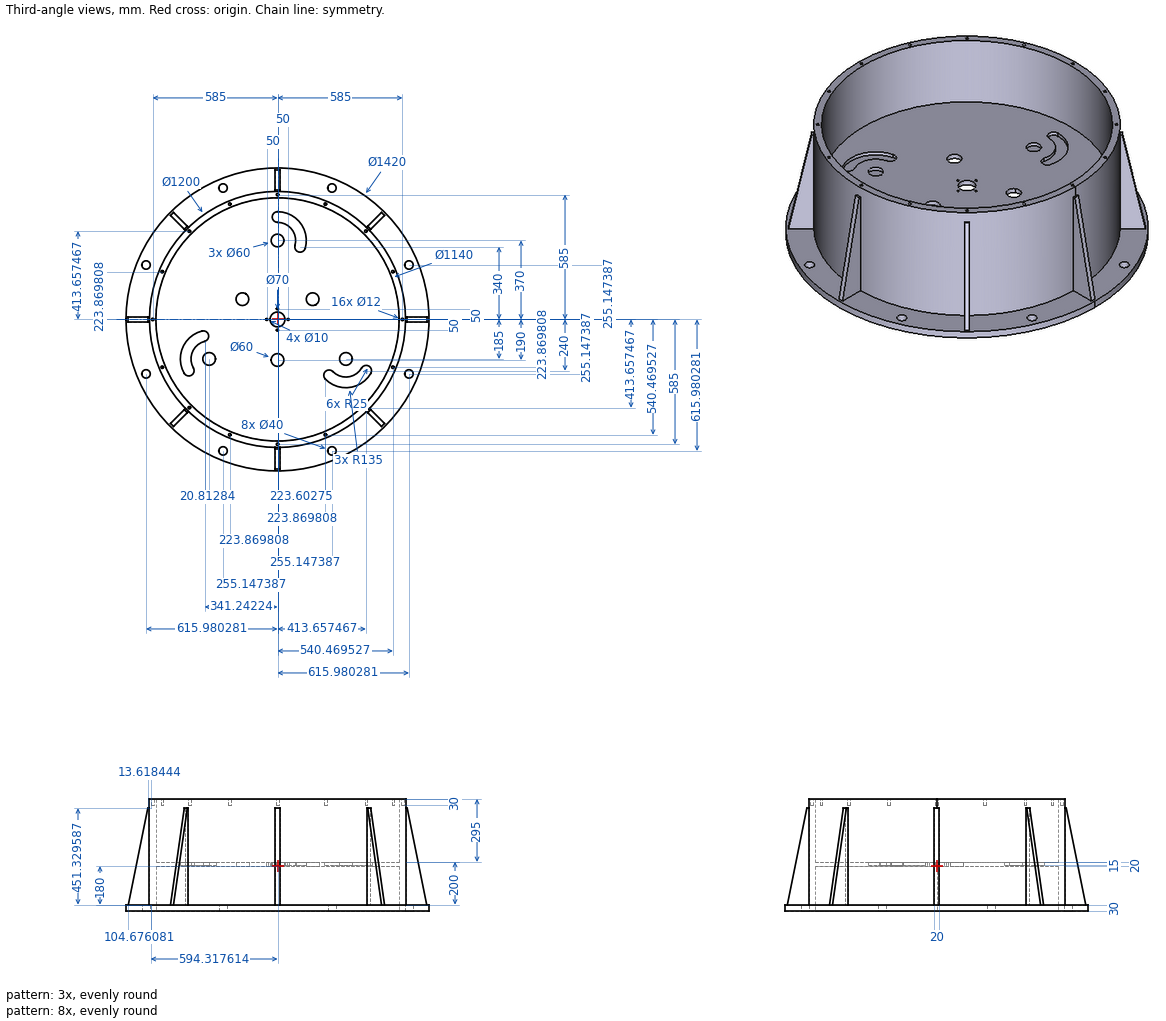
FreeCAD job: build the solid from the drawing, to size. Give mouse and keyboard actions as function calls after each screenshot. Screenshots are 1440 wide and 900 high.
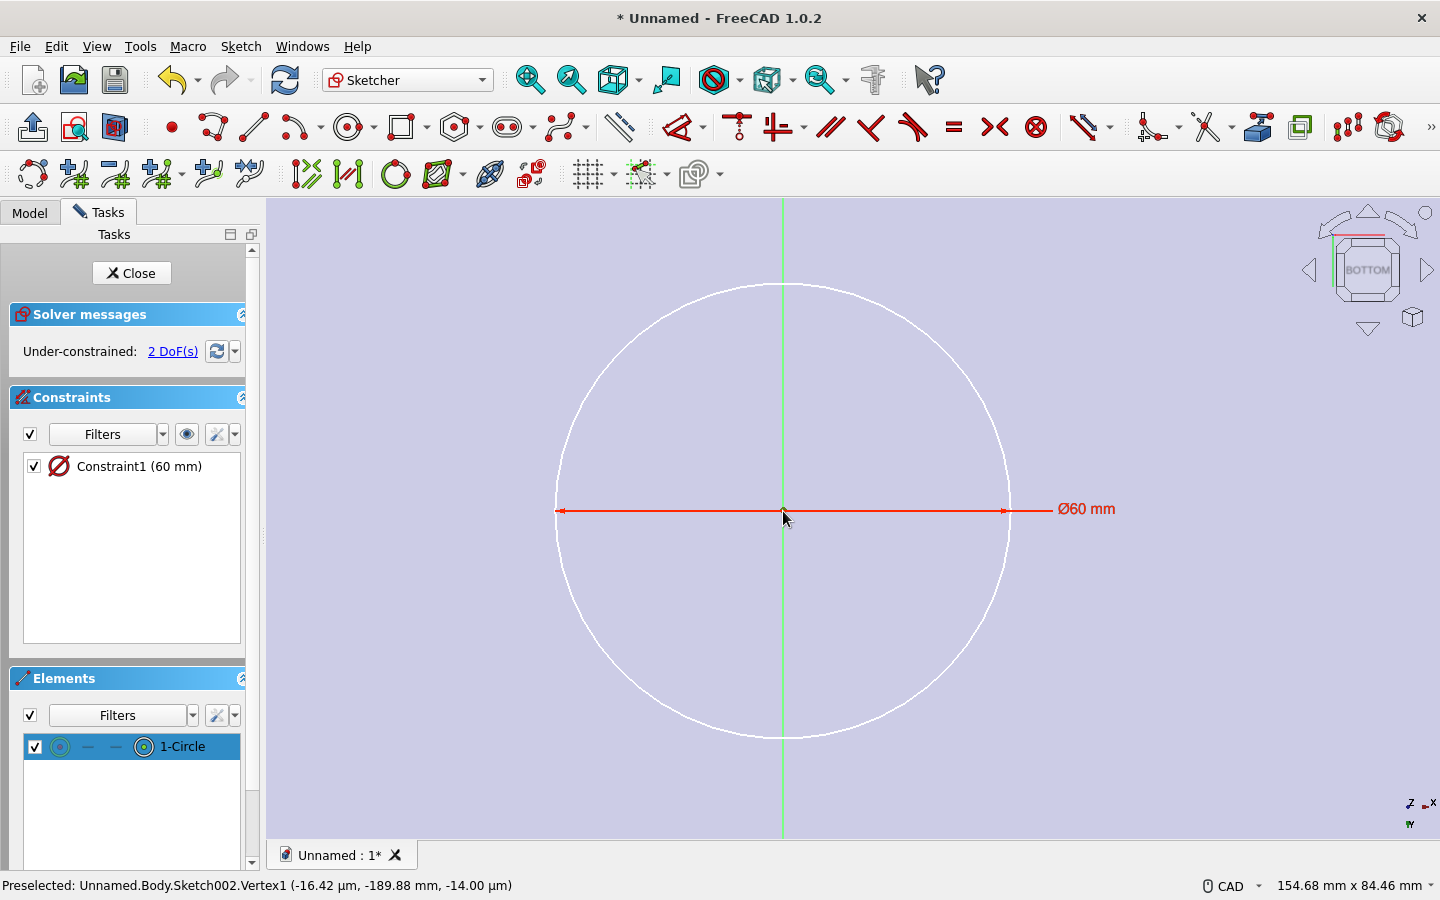
click(783, 769)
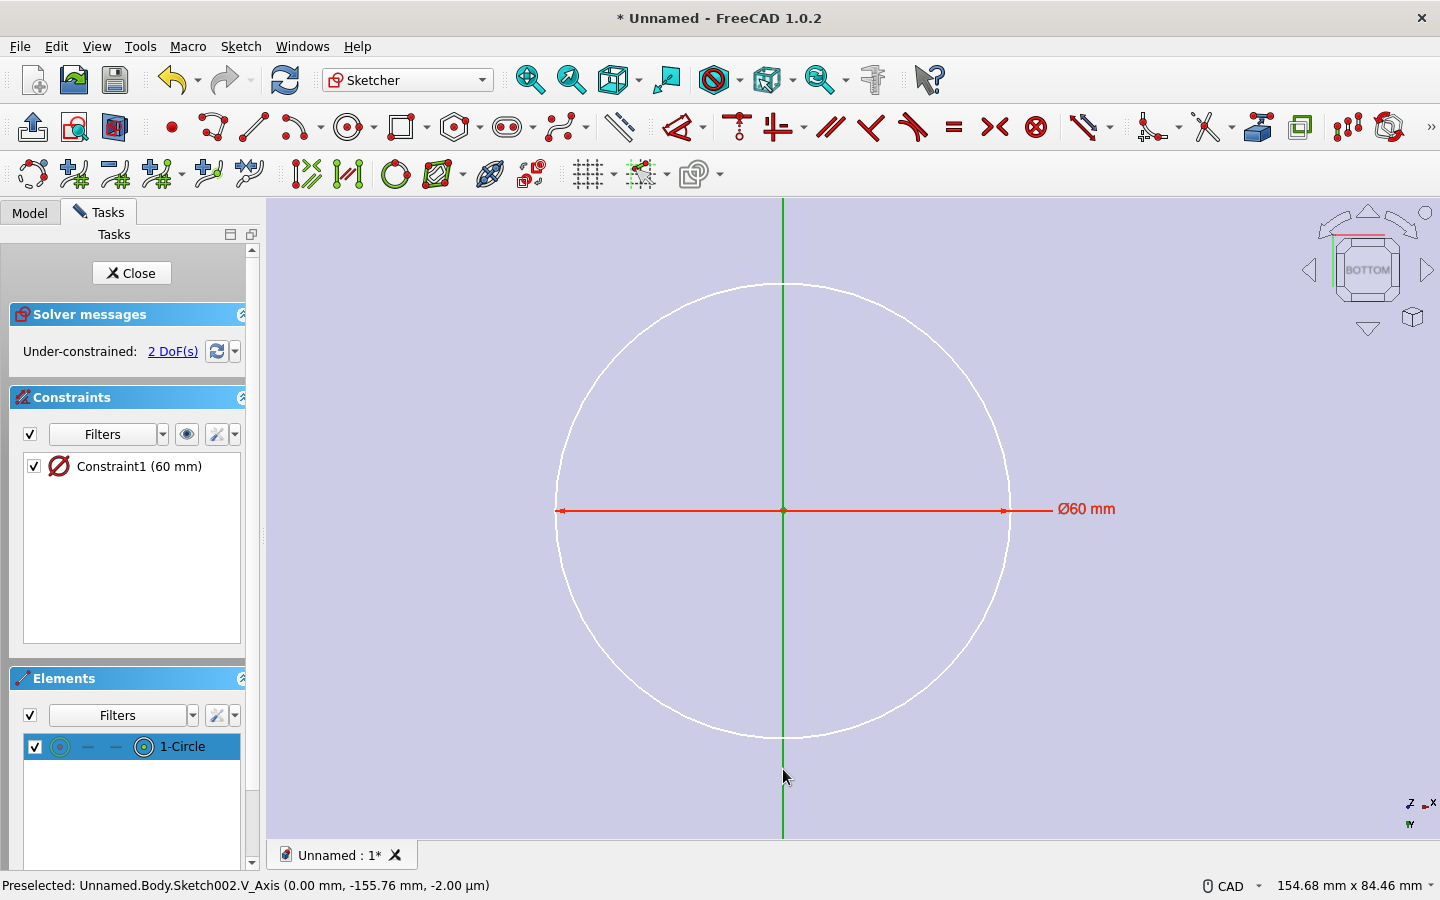
key(c)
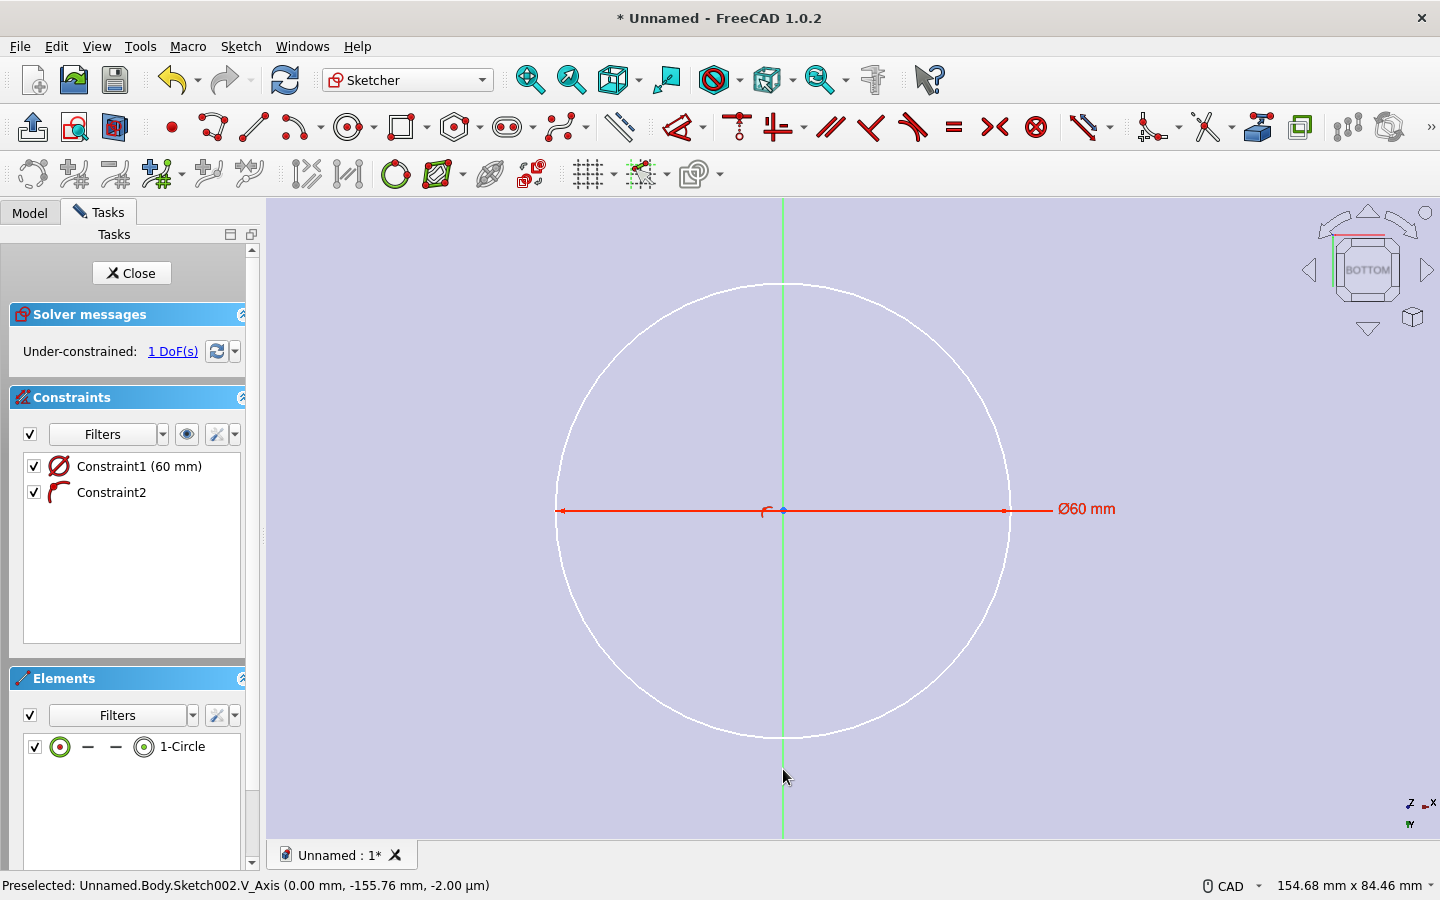
click(783, 511)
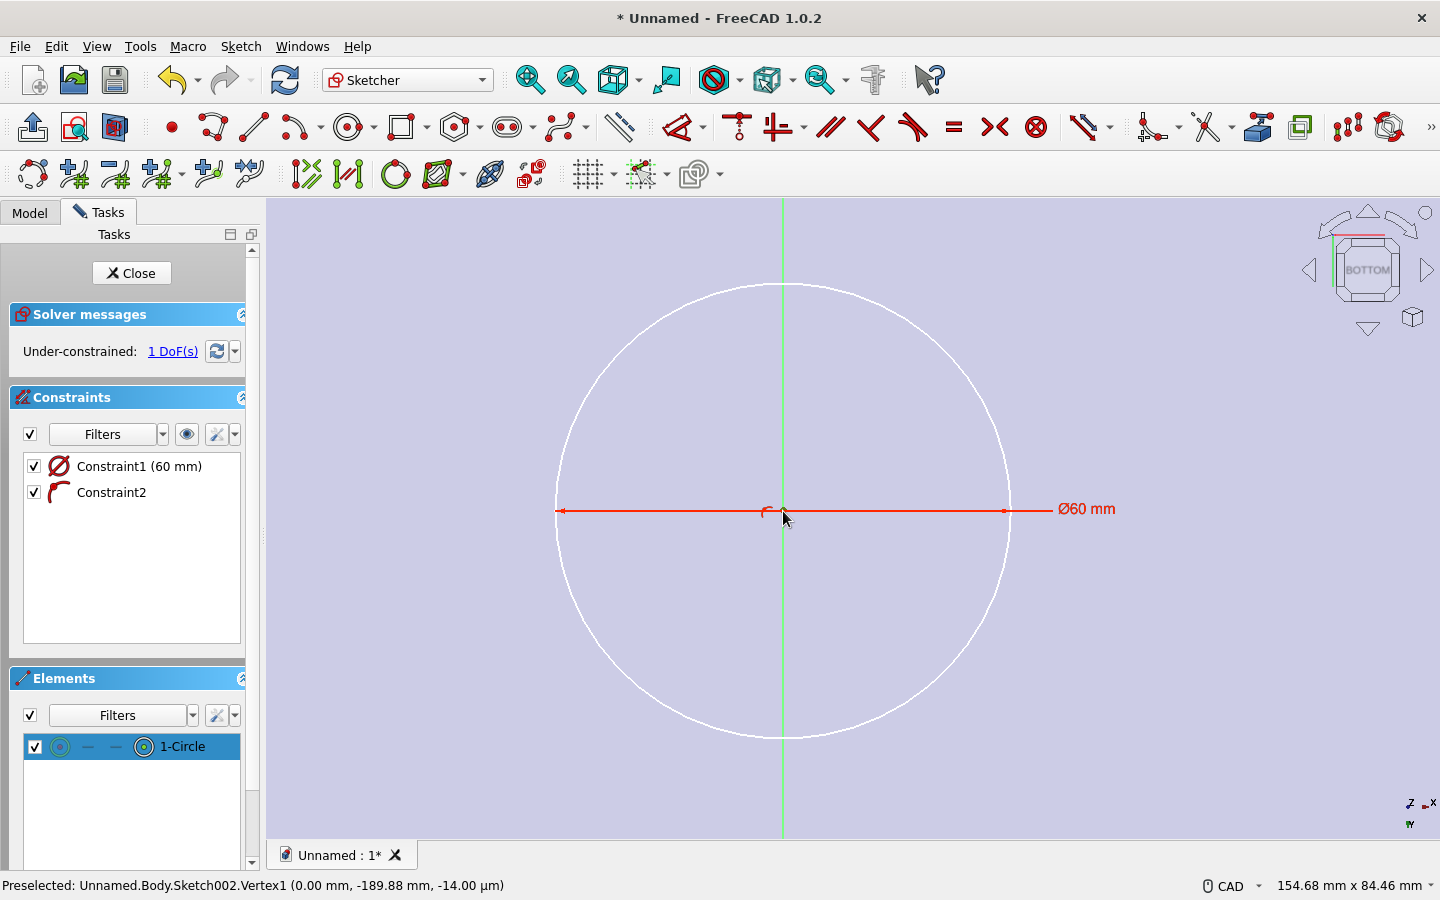
click(702, 128)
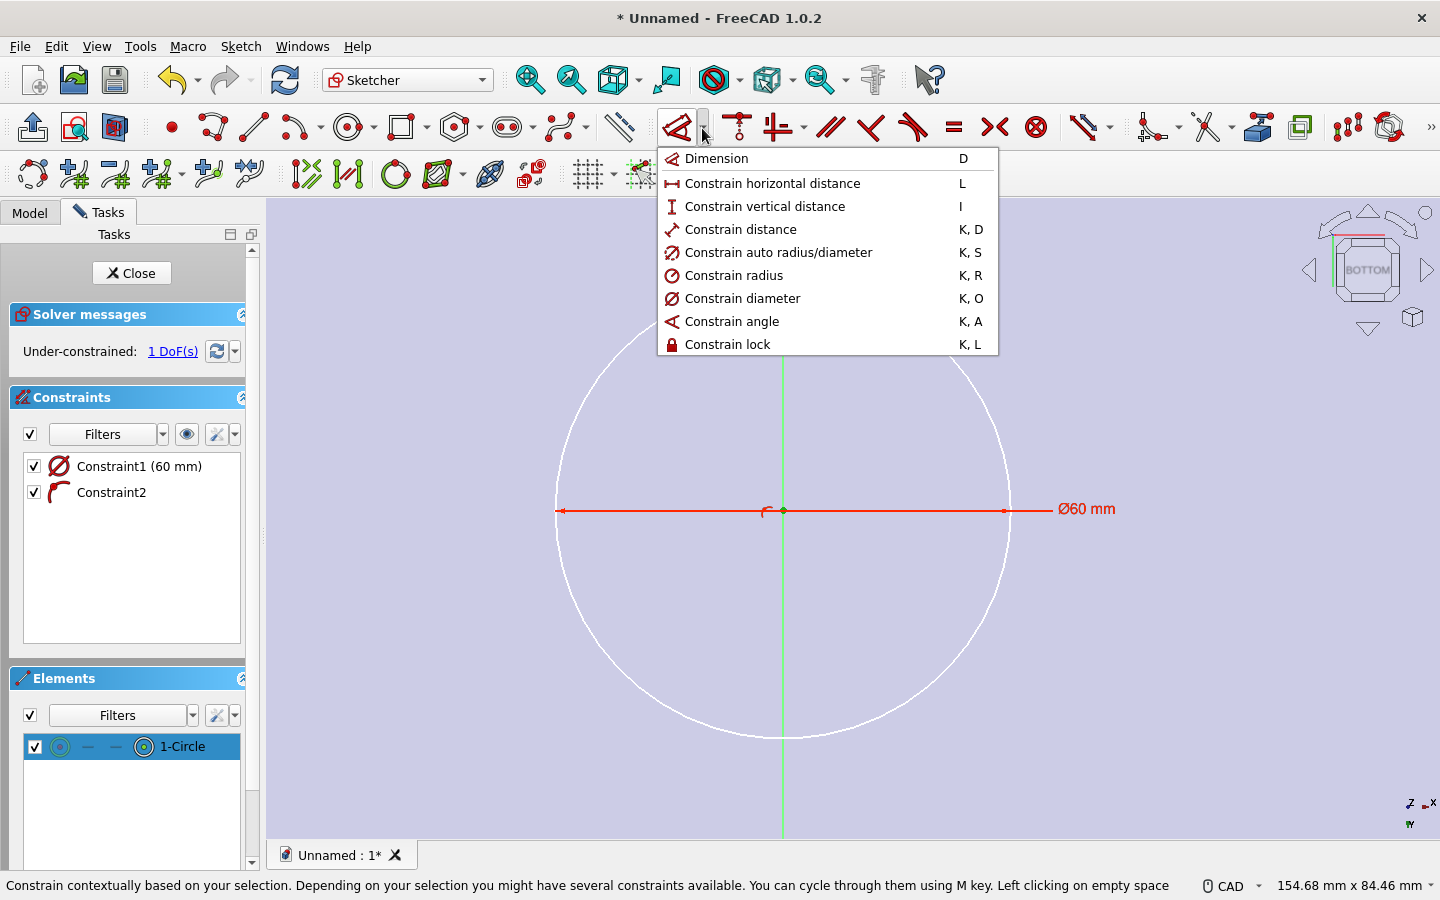
click(828, 206)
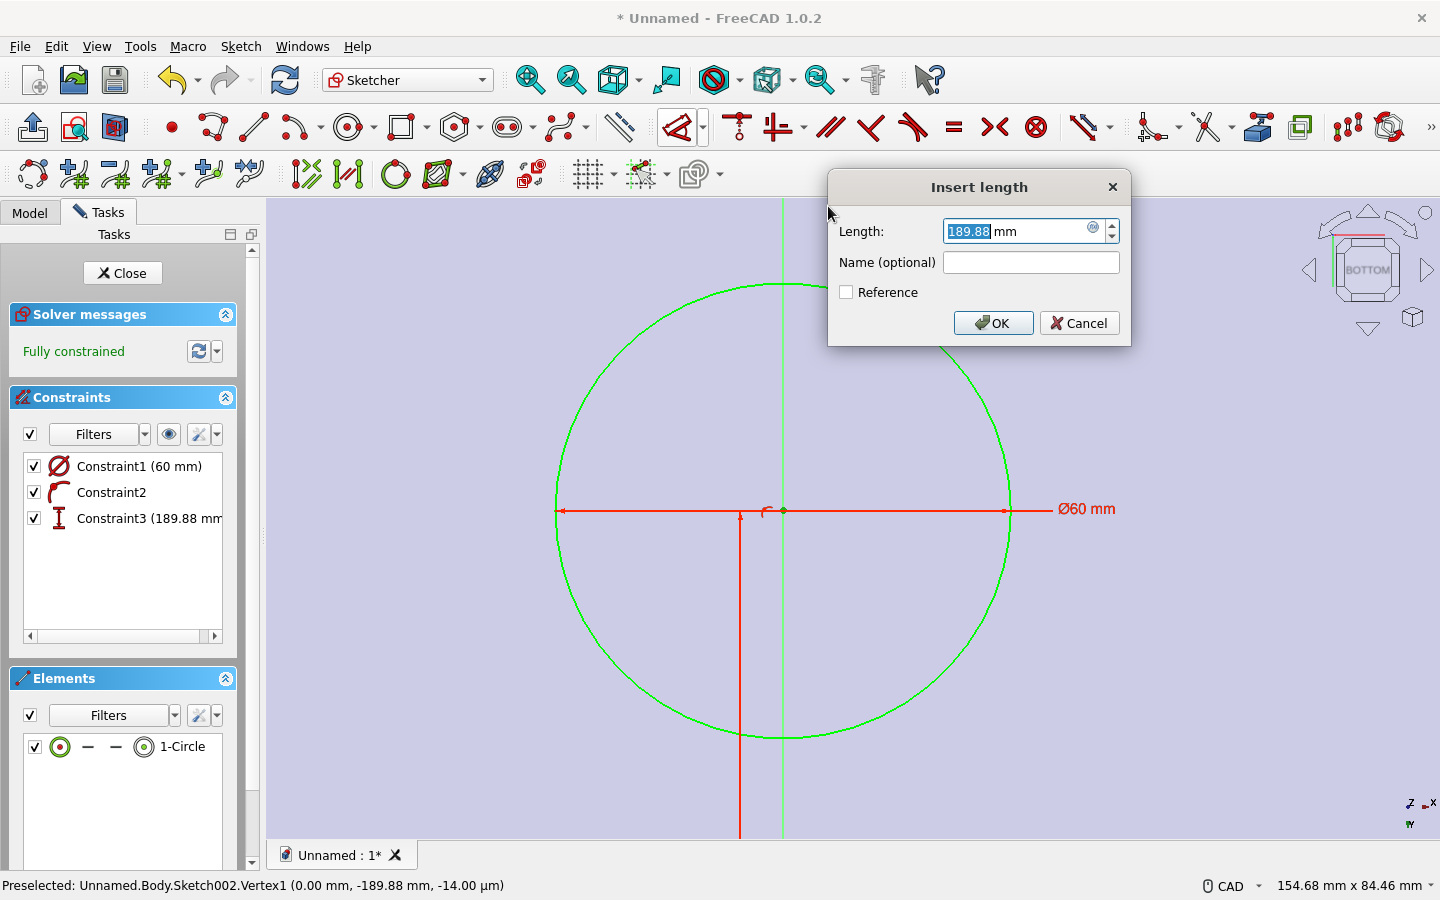
text(190)
key(Return)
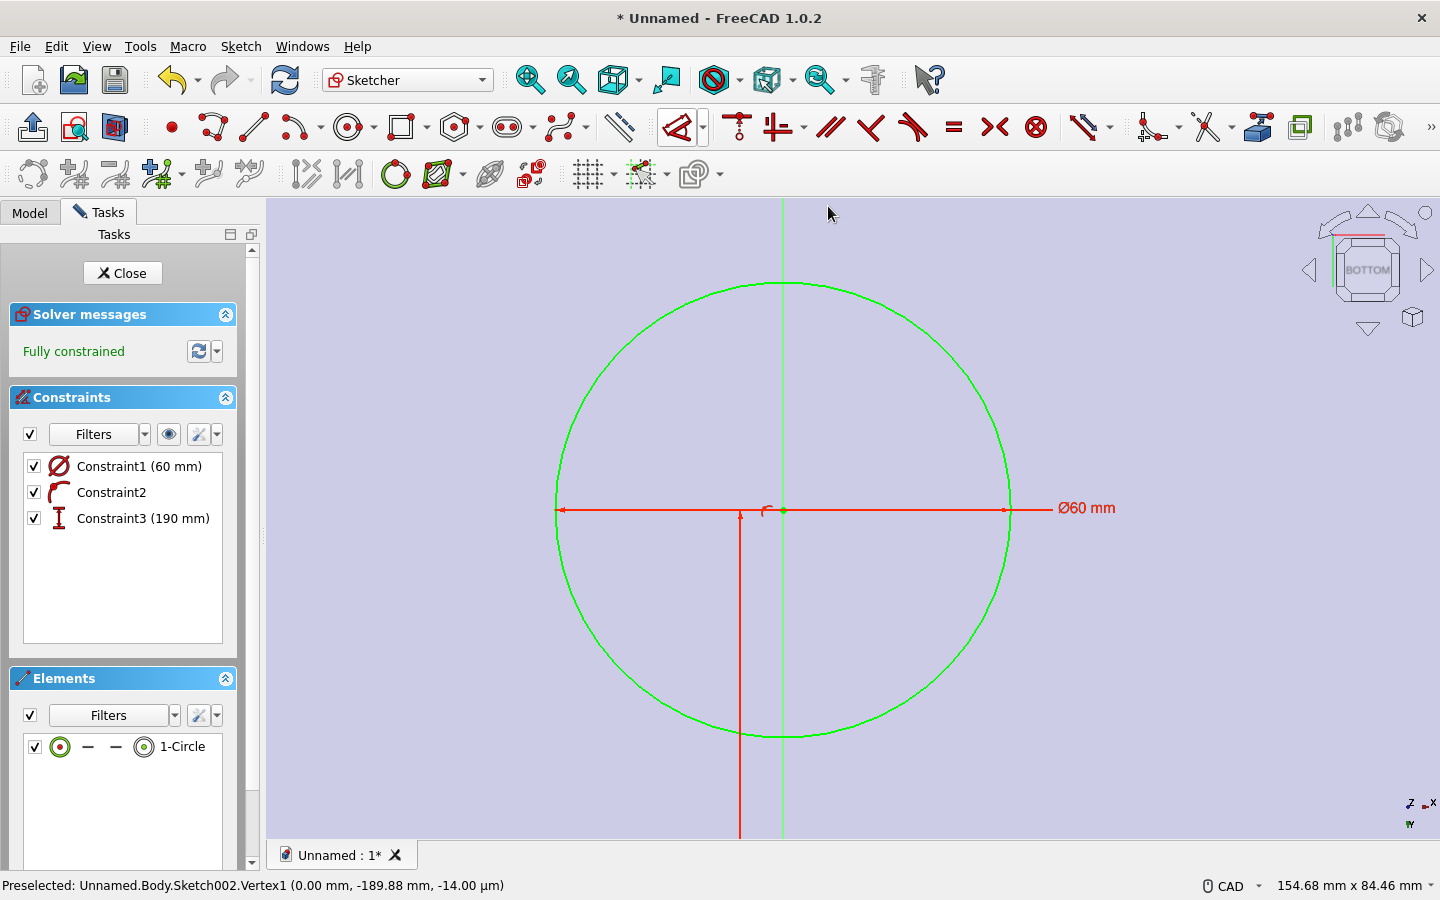
click(123, 273)